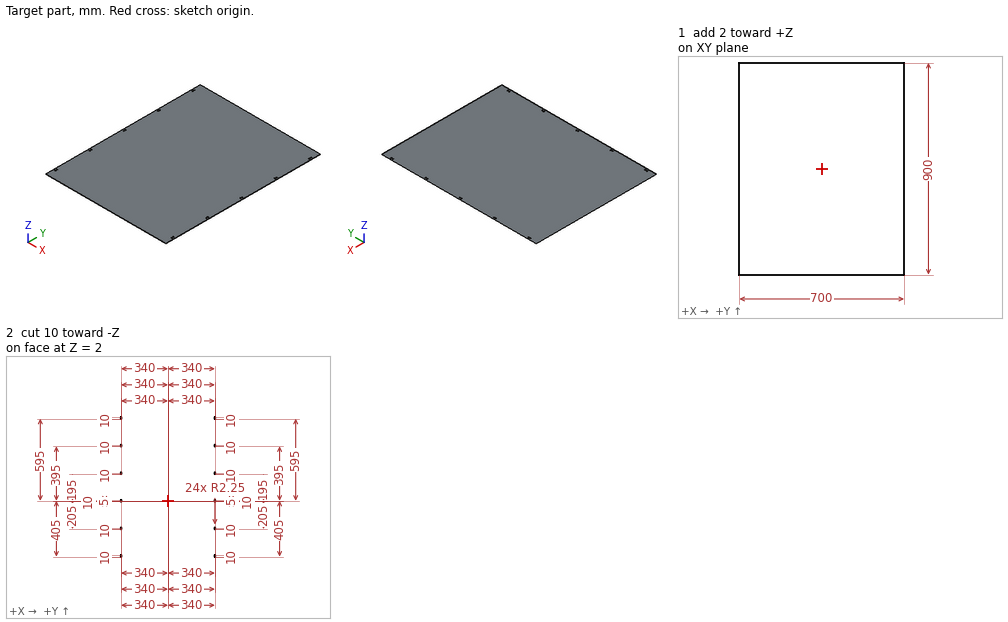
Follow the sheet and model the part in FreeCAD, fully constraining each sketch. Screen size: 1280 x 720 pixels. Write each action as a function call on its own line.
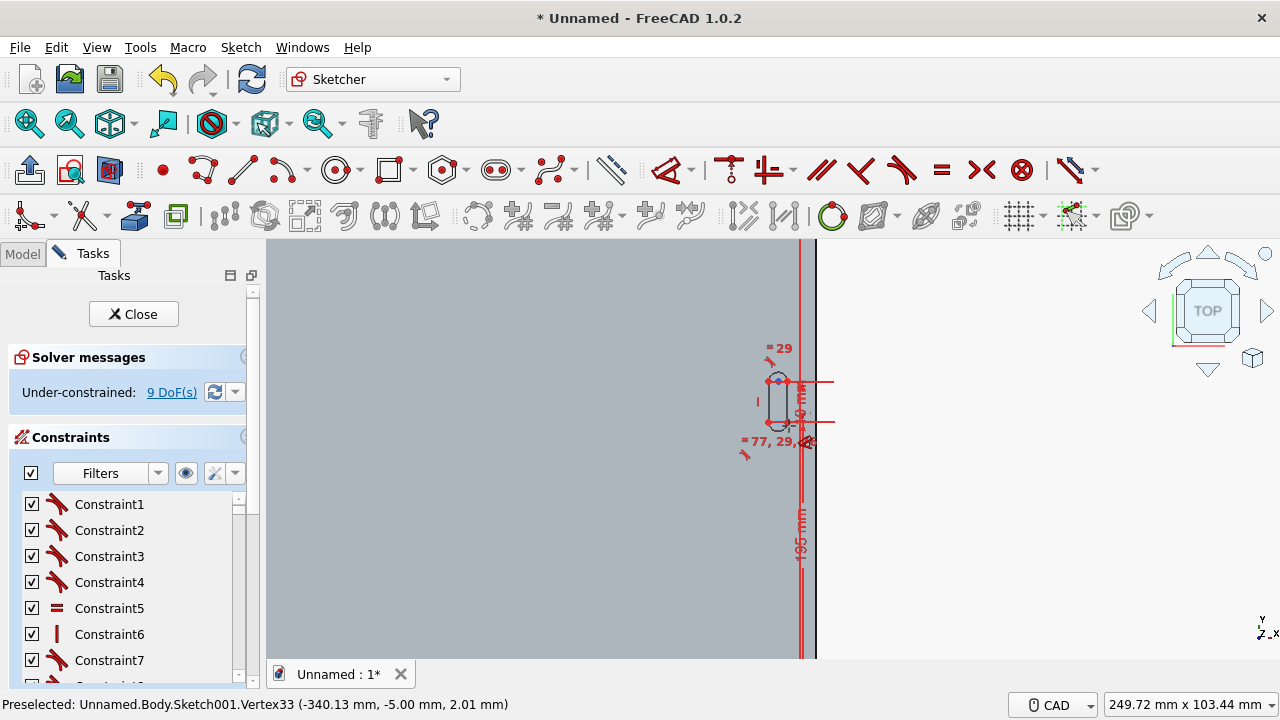
click(778, 422)
click(536, 388)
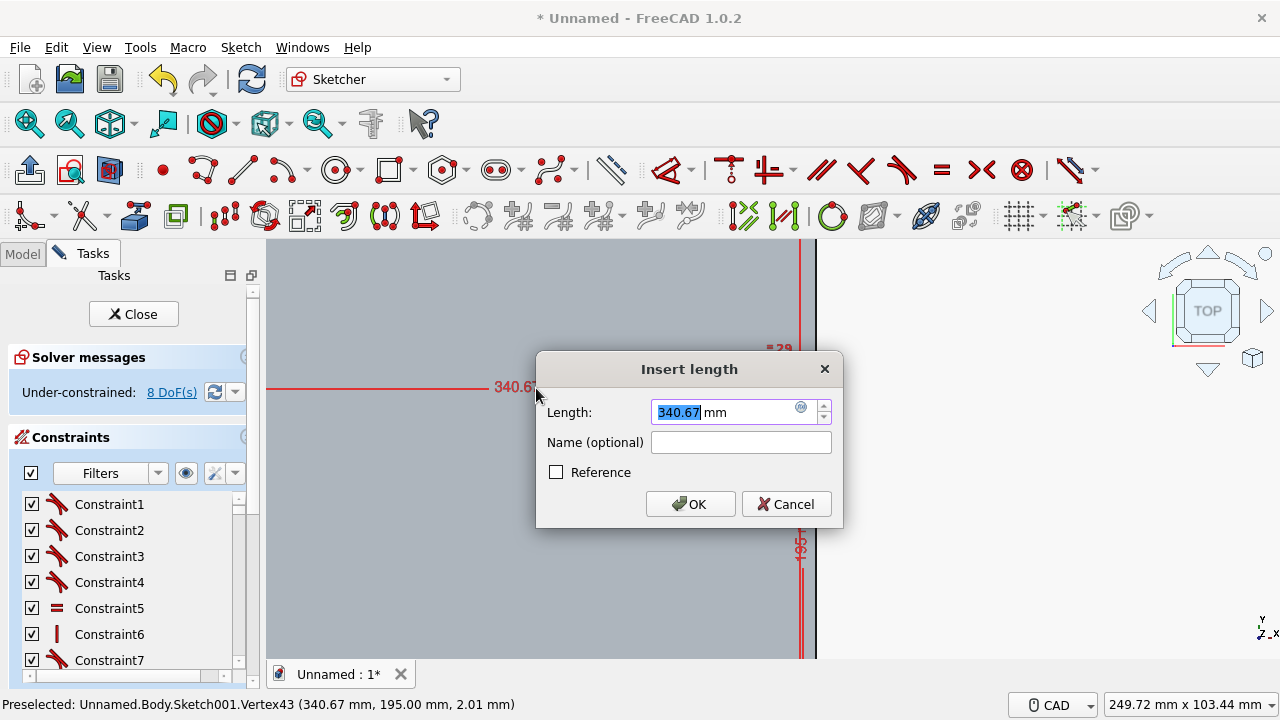
text(340)
key(Return)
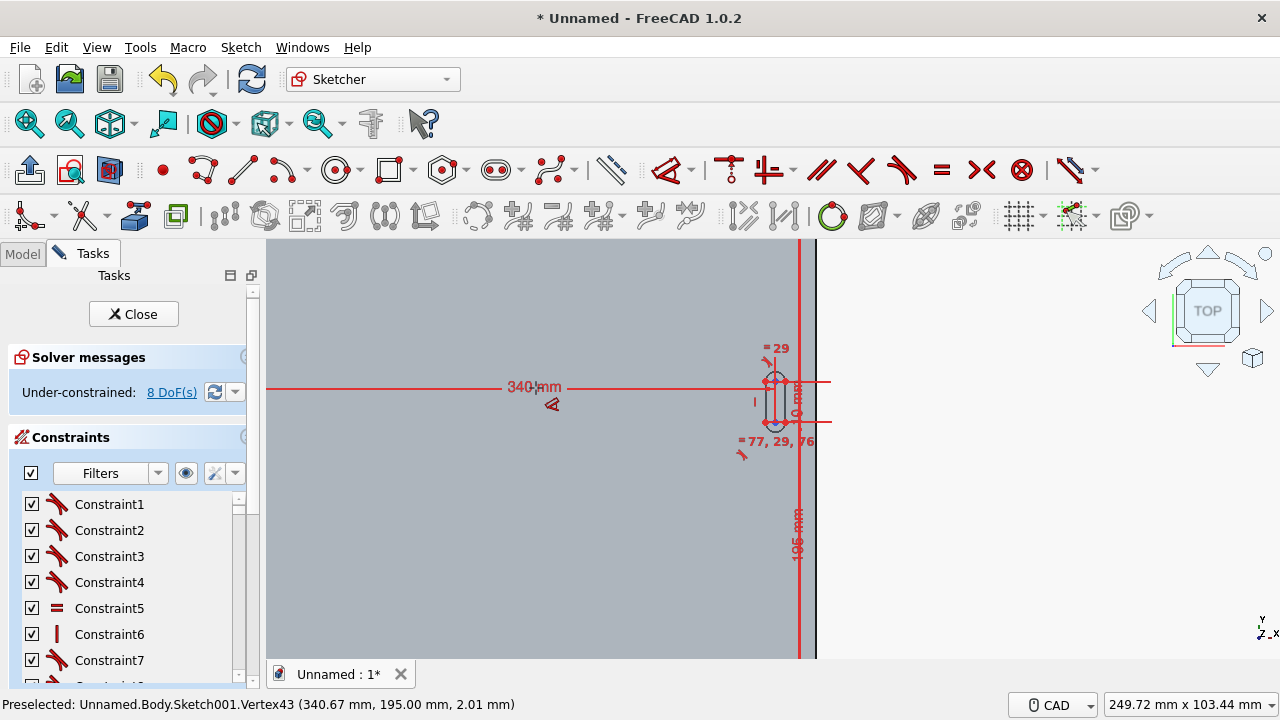
scroll(789, 426, down, 14)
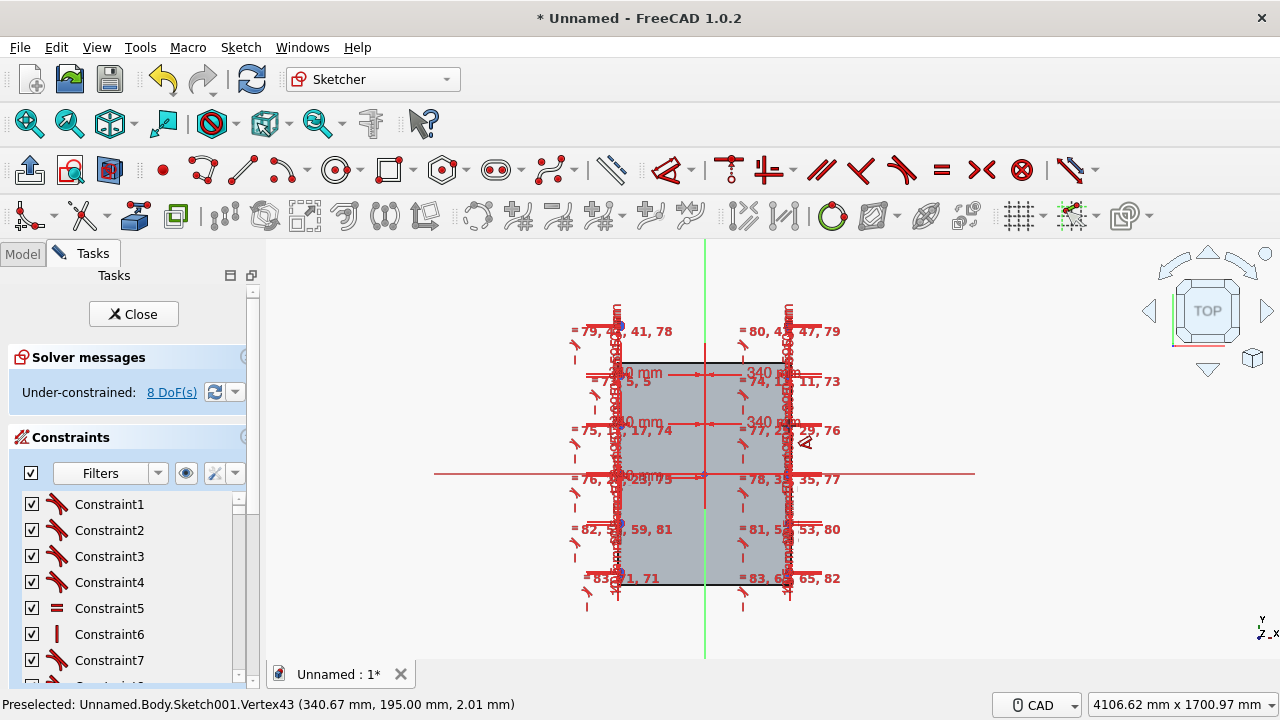
scroll(789, 476, up, 14)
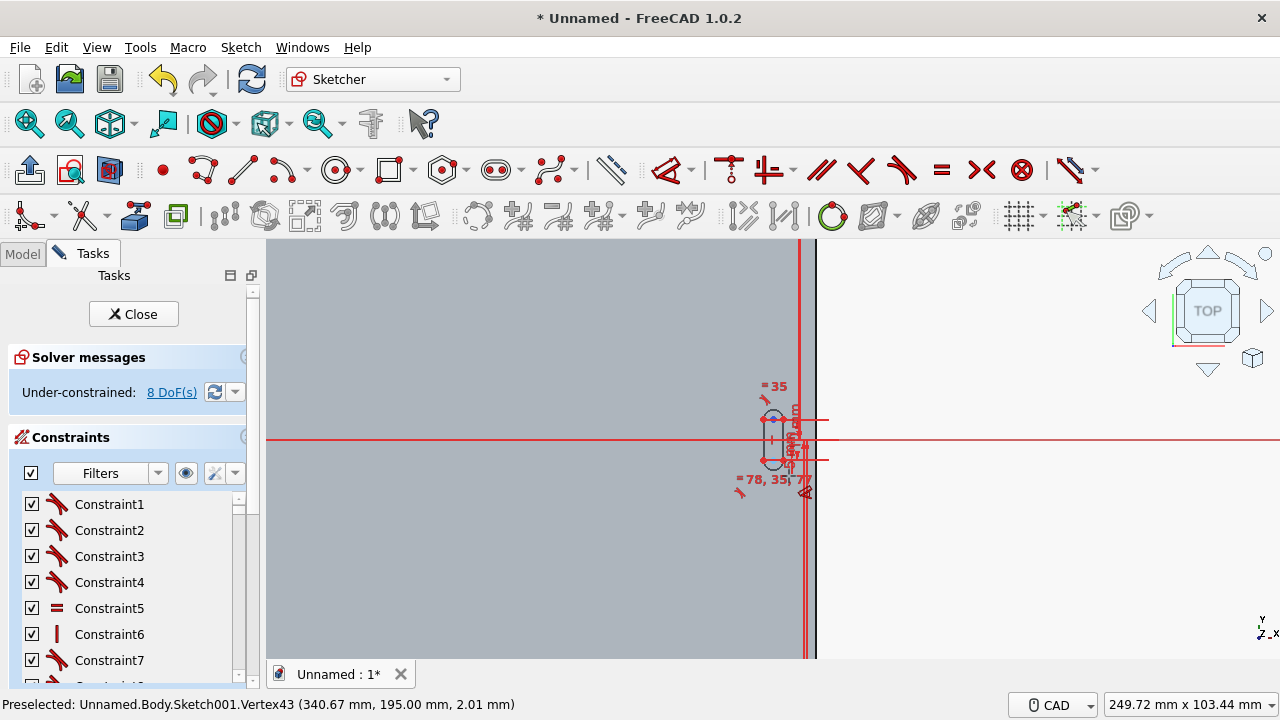
click(773, 460)
click(534, 494)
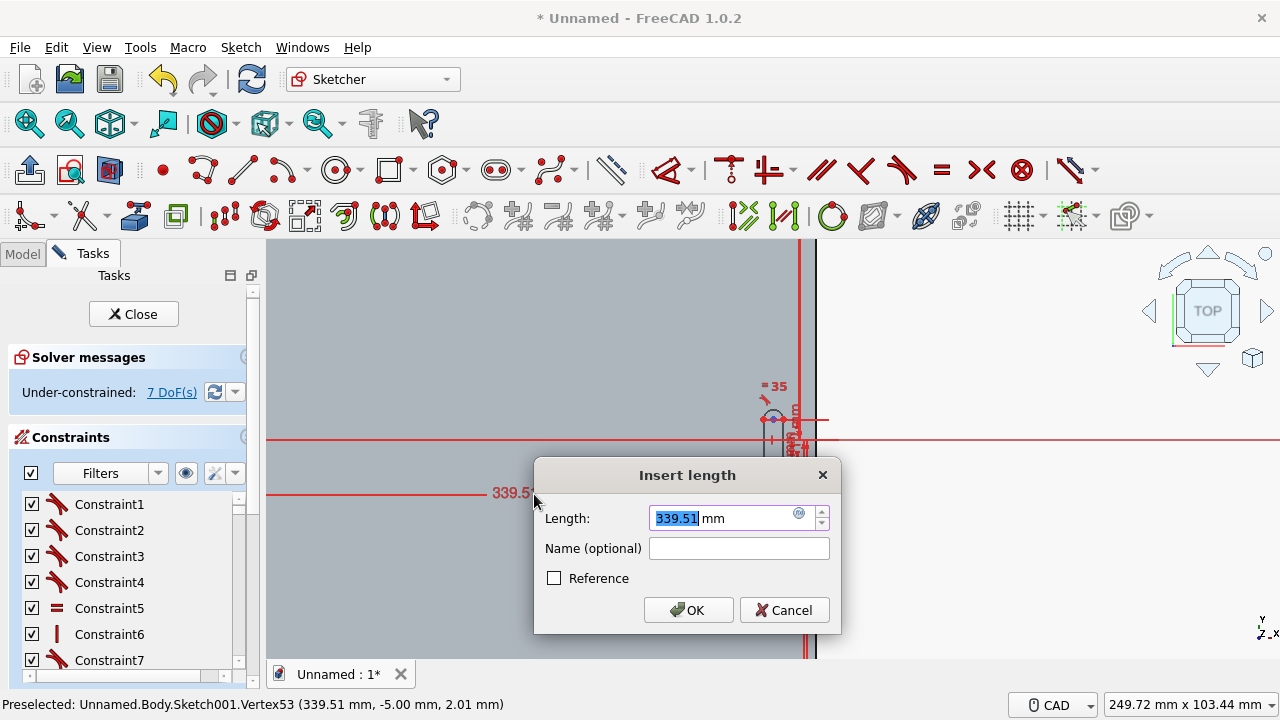
text(340)
key(Return)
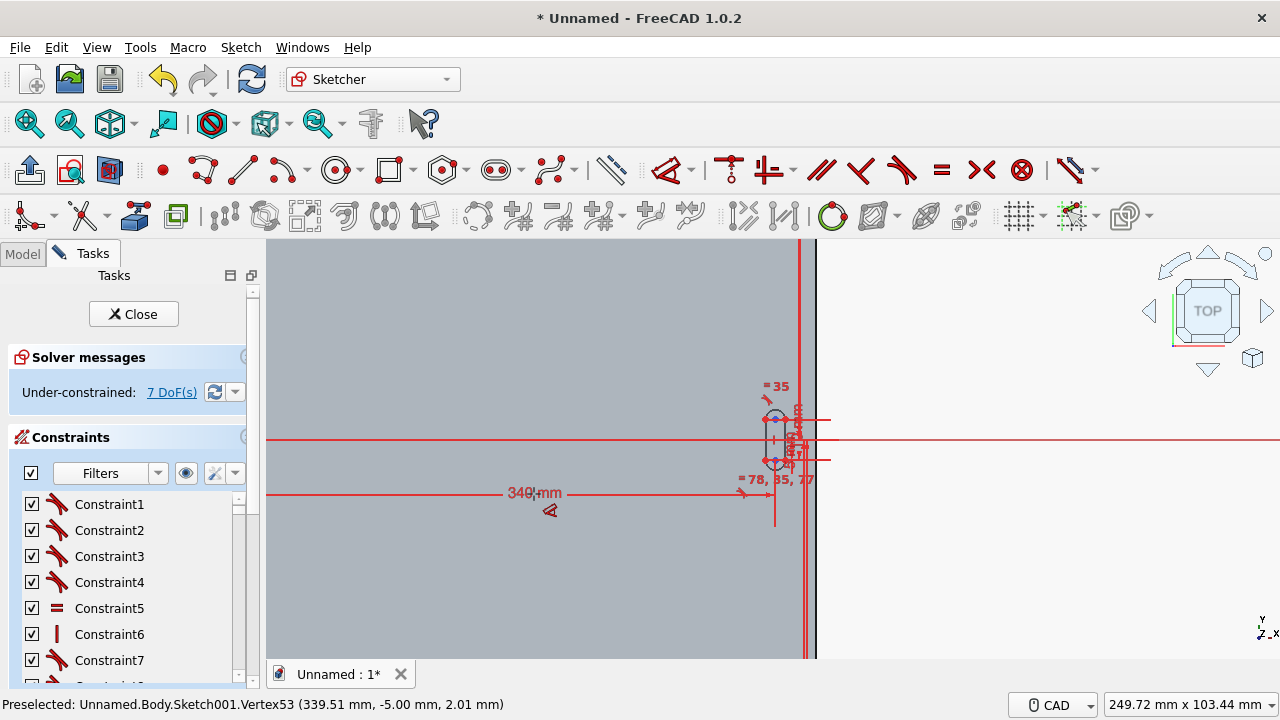
scroll(789, 476, down, 14)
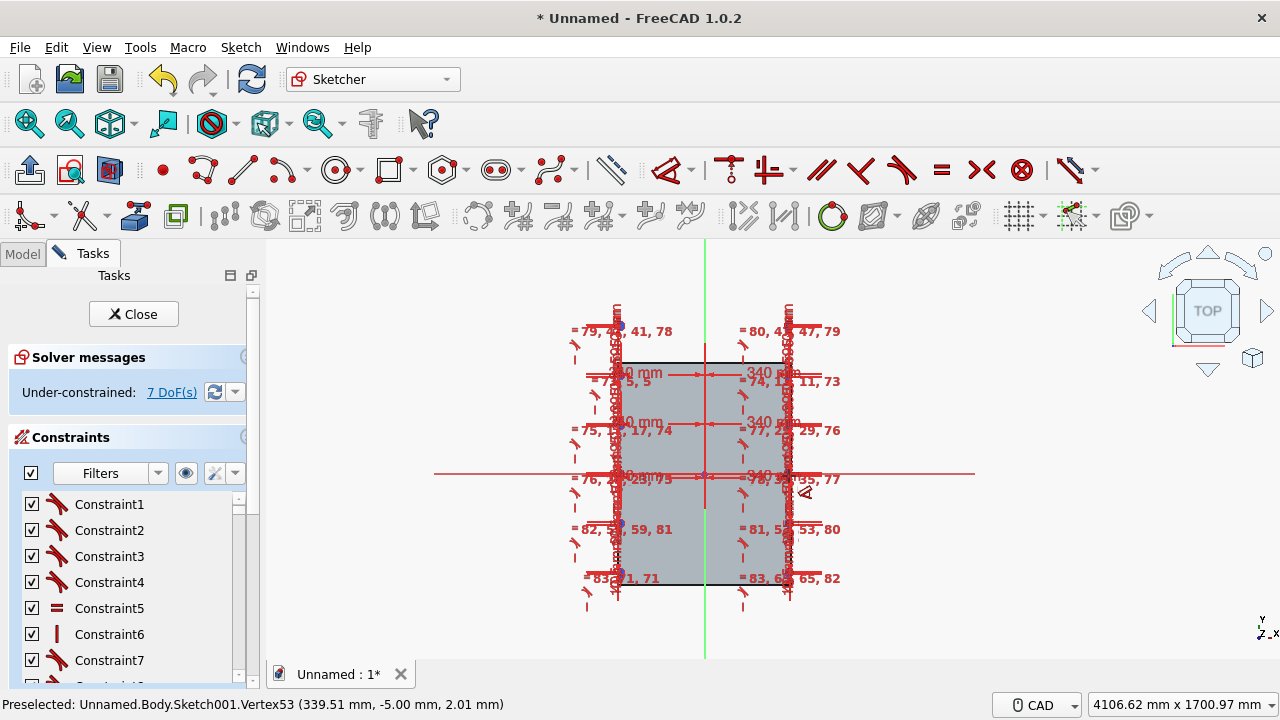
scroll(621, 327, up, 14)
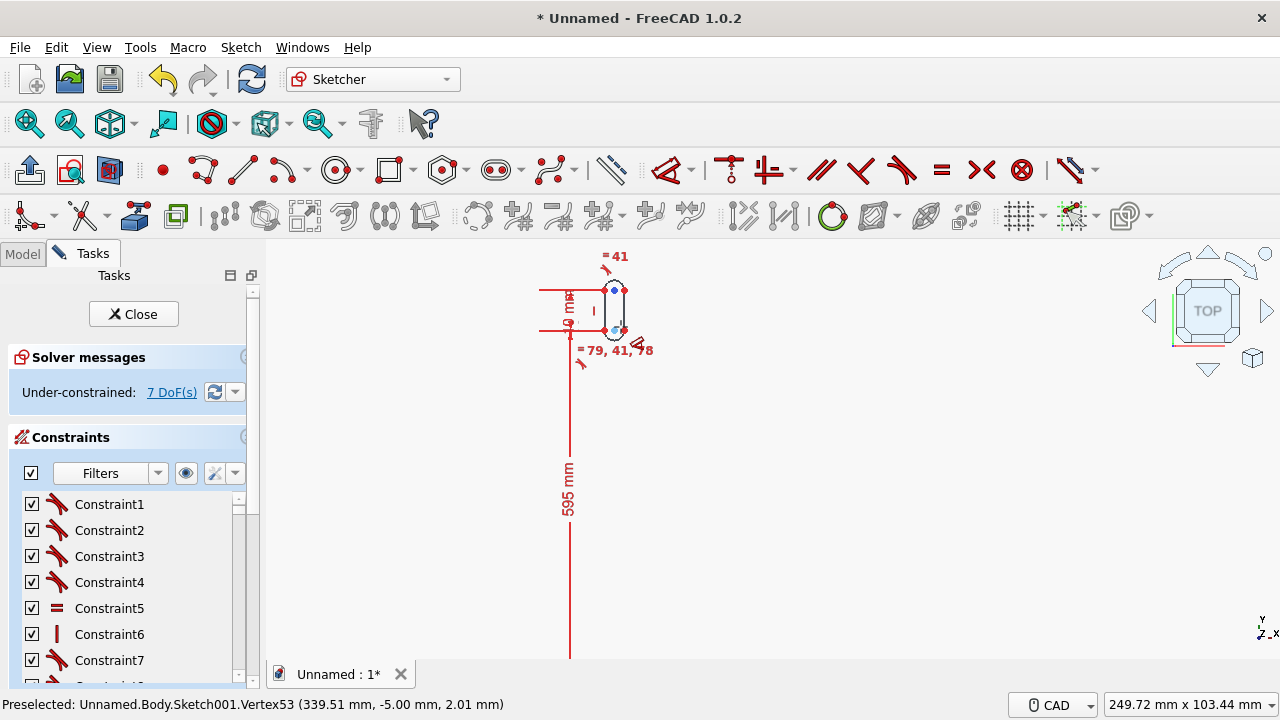
click(614, 331)
click(865, 297)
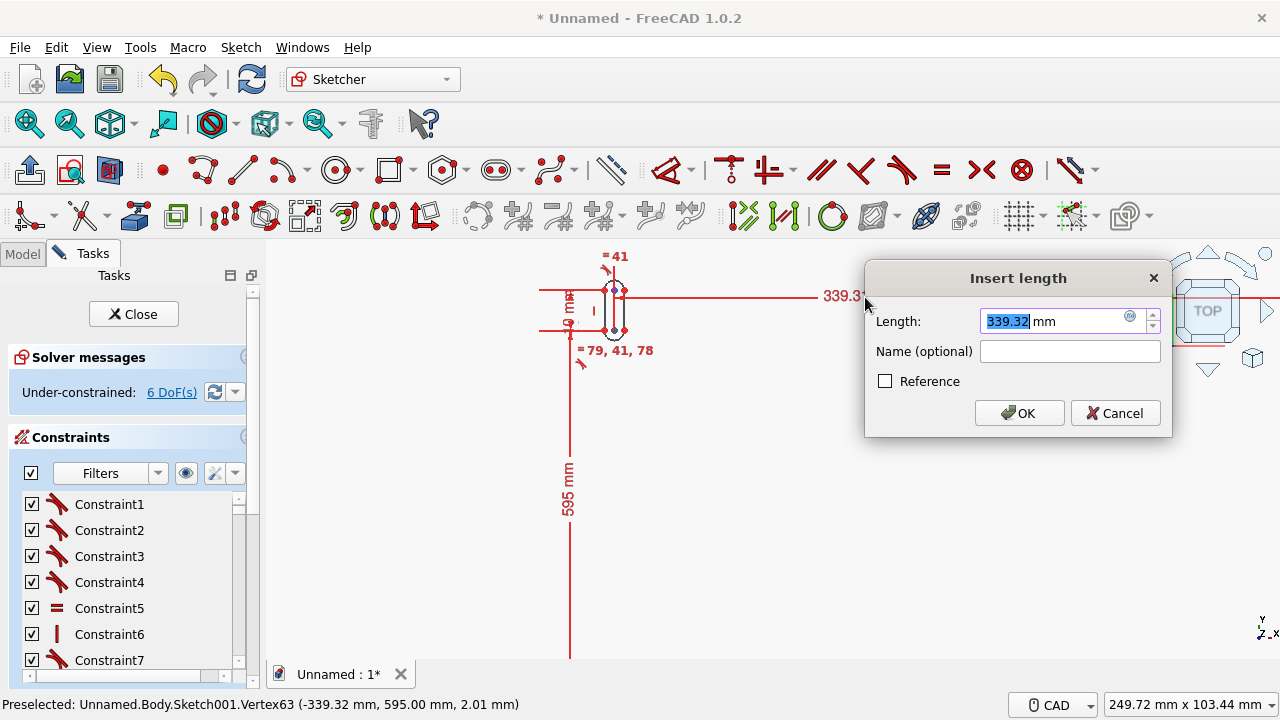
text(340)
key(Return)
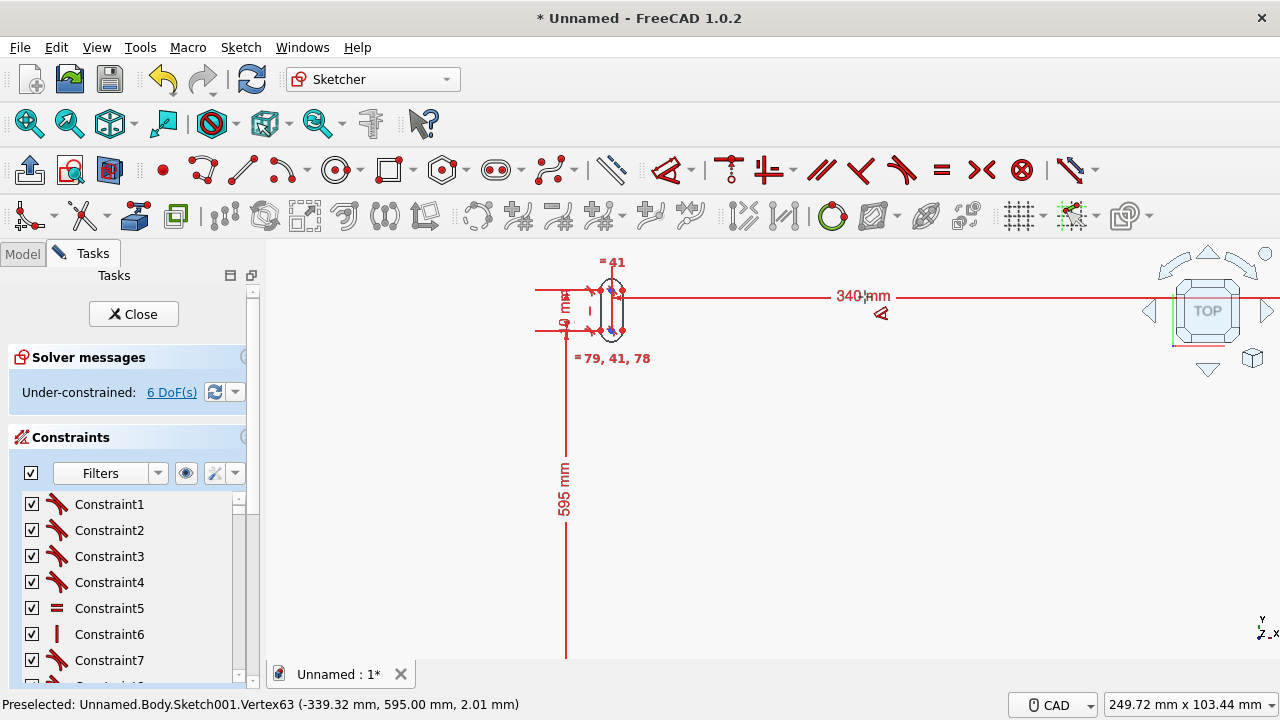
scroll(621, 327, down, 14)